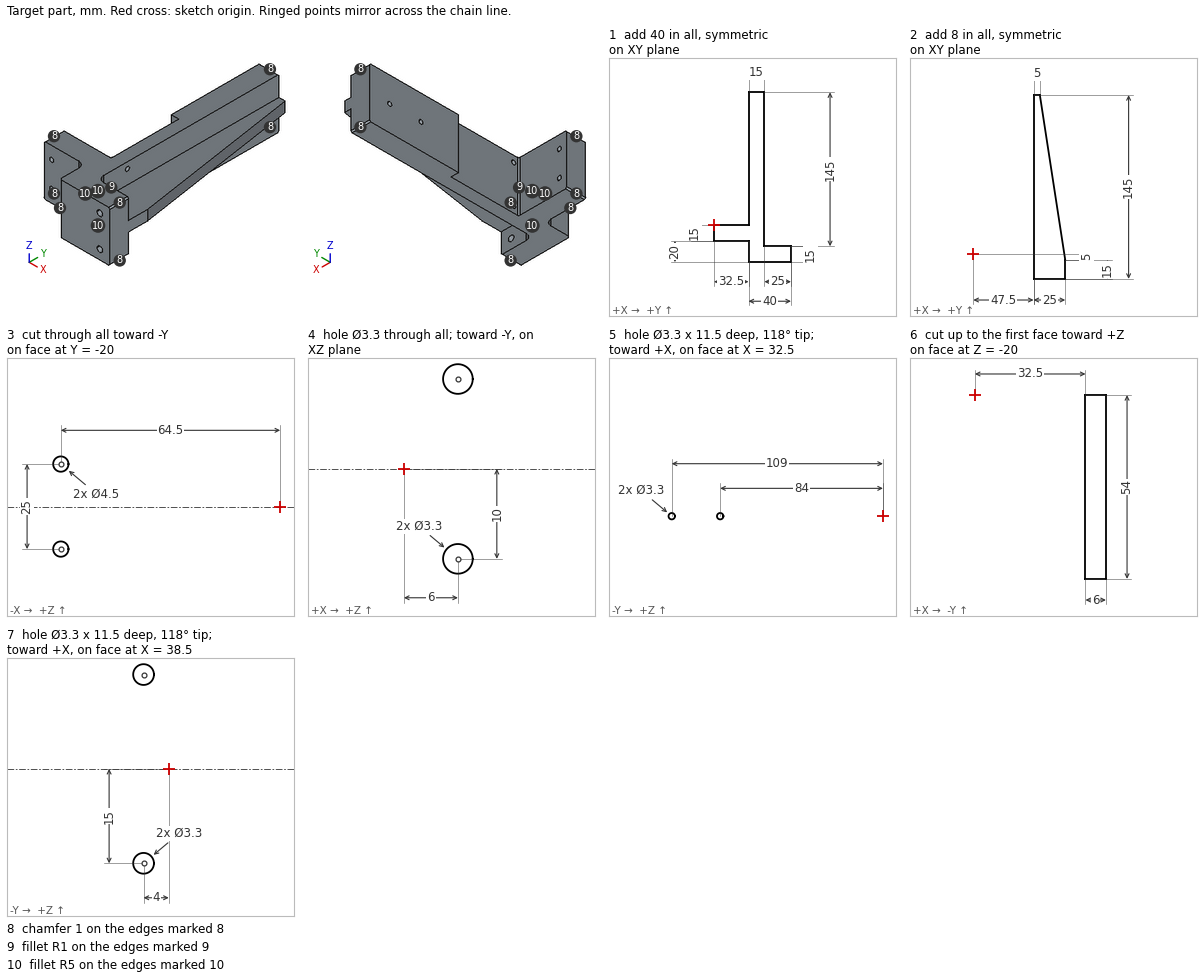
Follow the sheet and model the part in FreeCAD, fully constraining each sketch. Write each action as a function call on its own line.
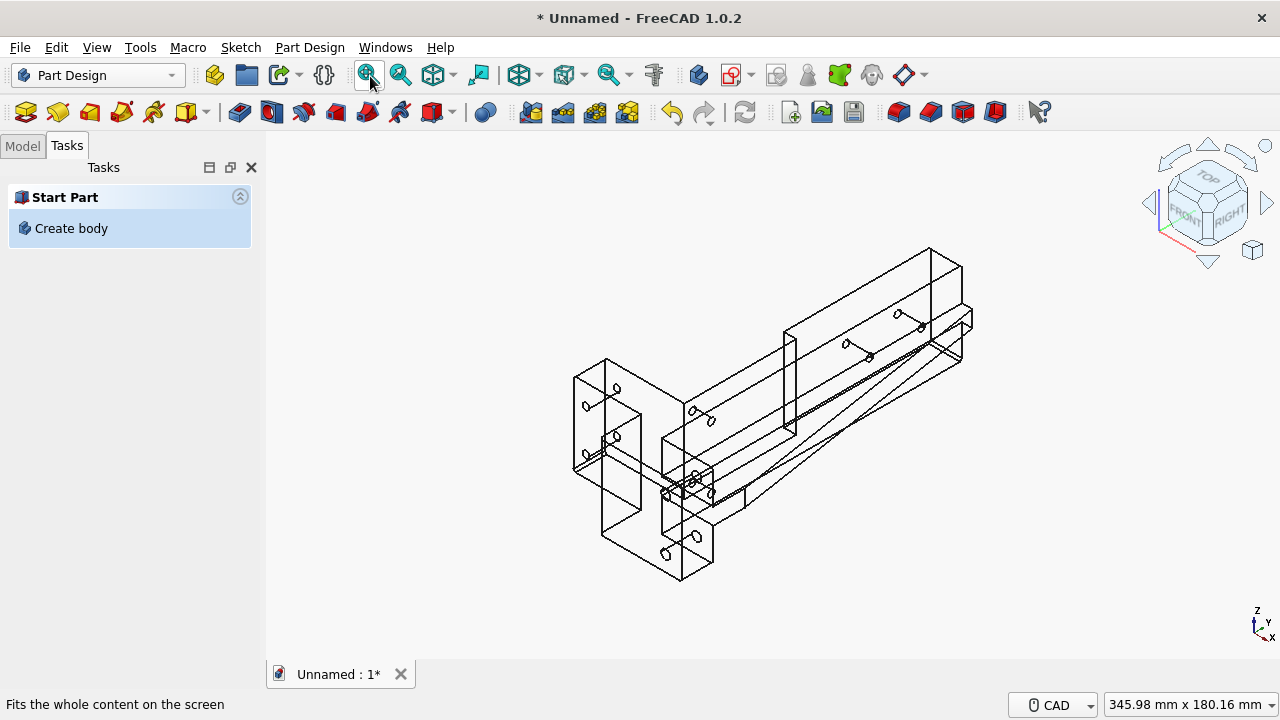
click(684, 441)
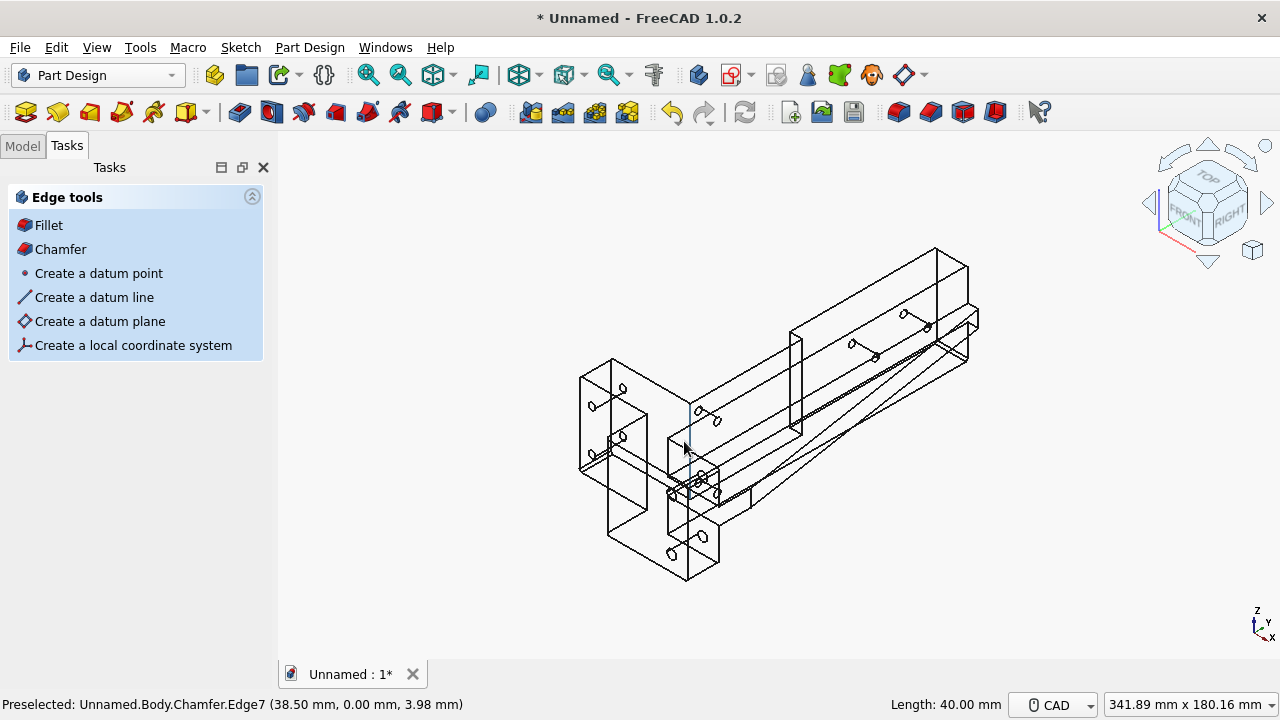
key(v)
key(1)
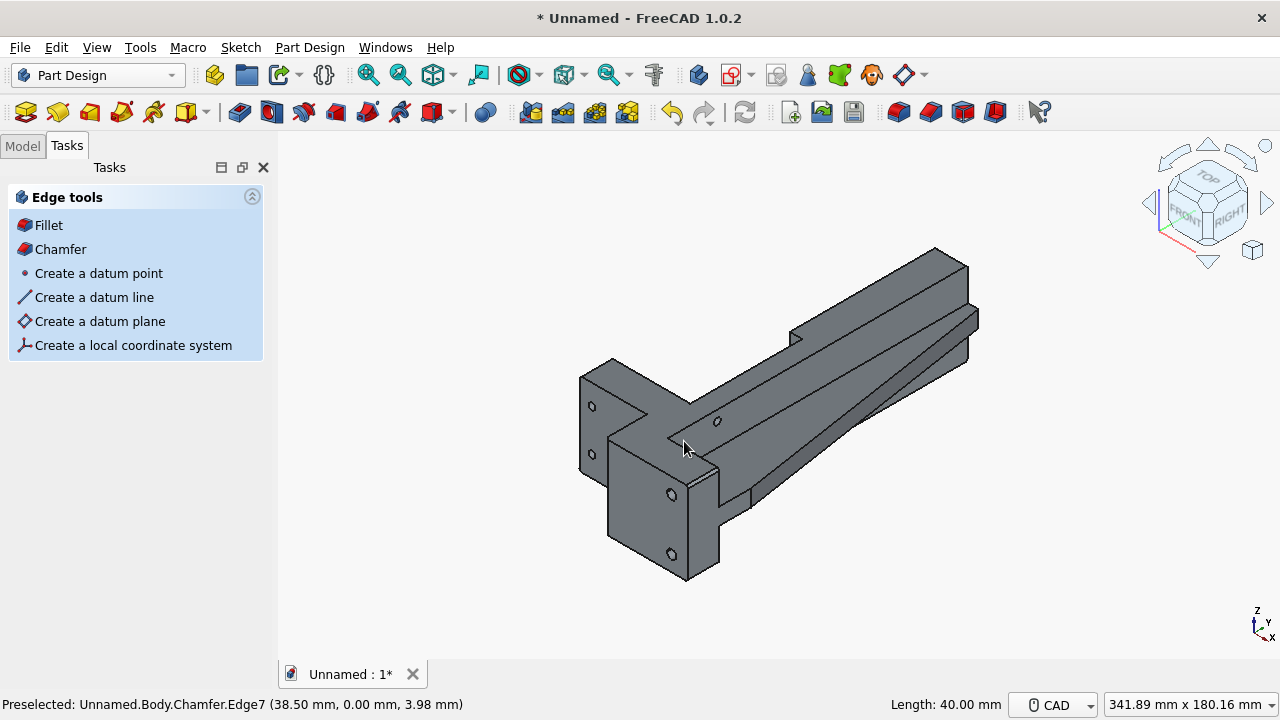
click(900, 112)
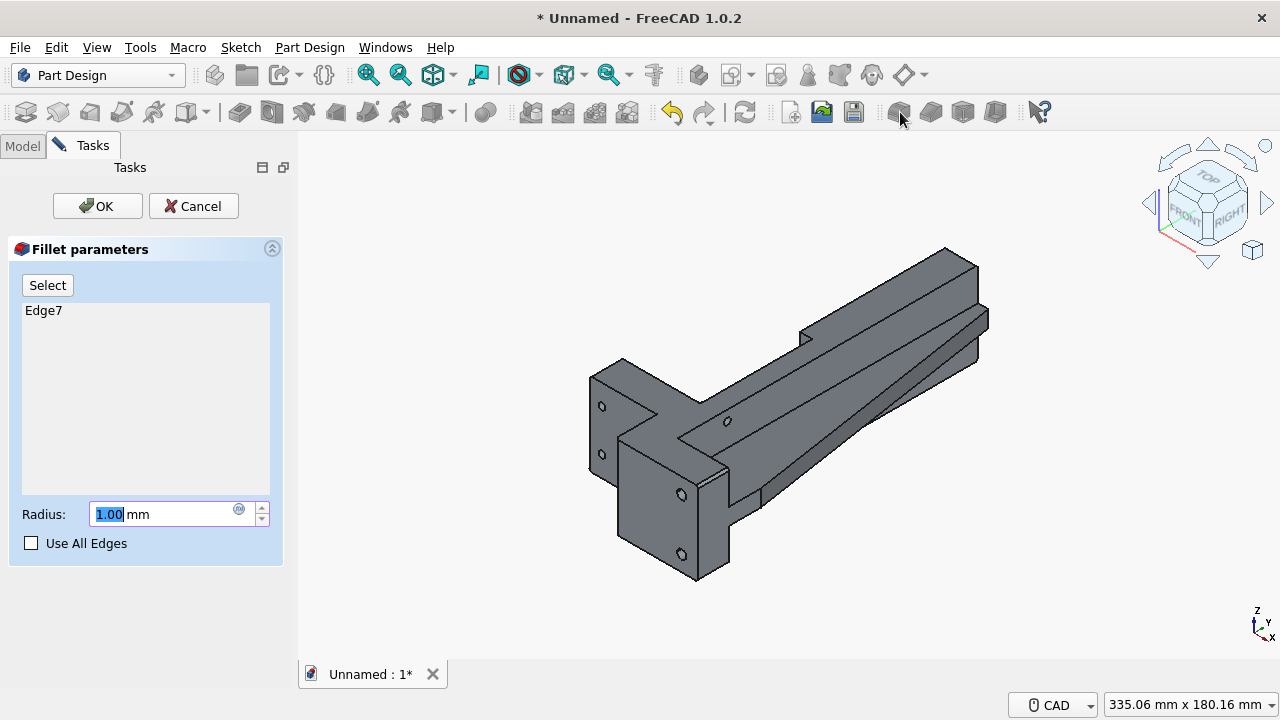
text(1)
key(Tab)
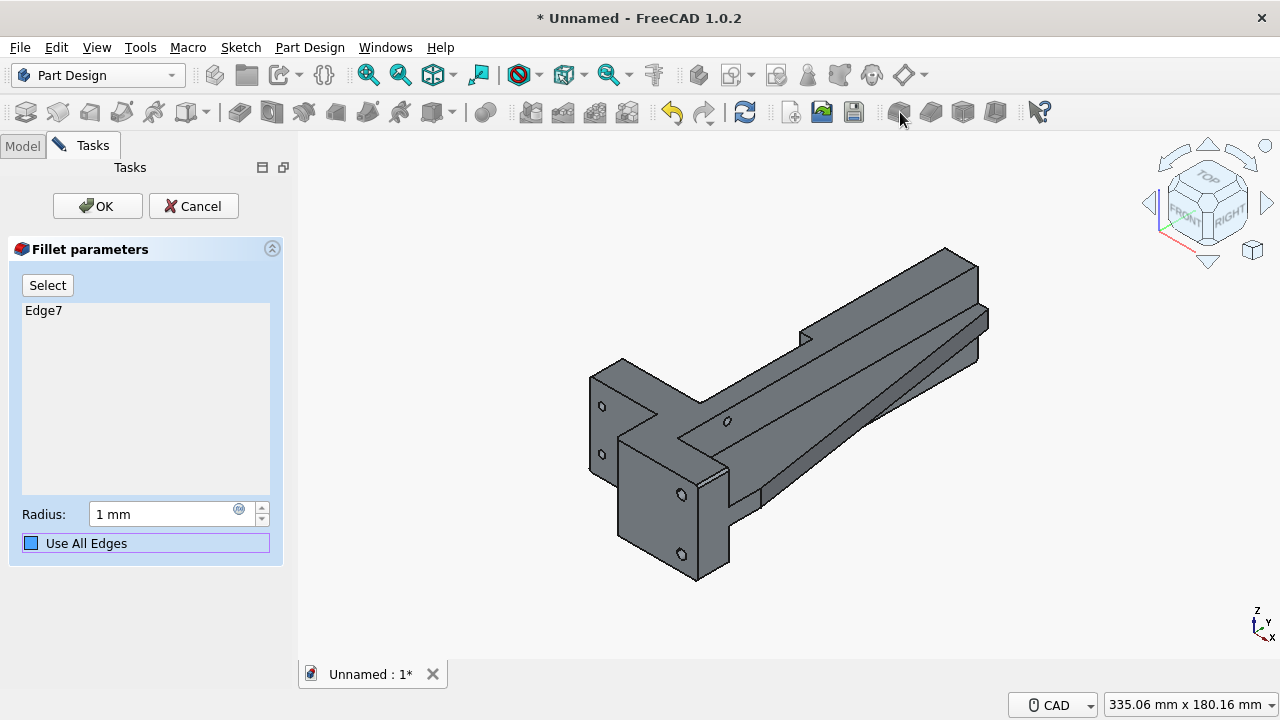
click(98, 206)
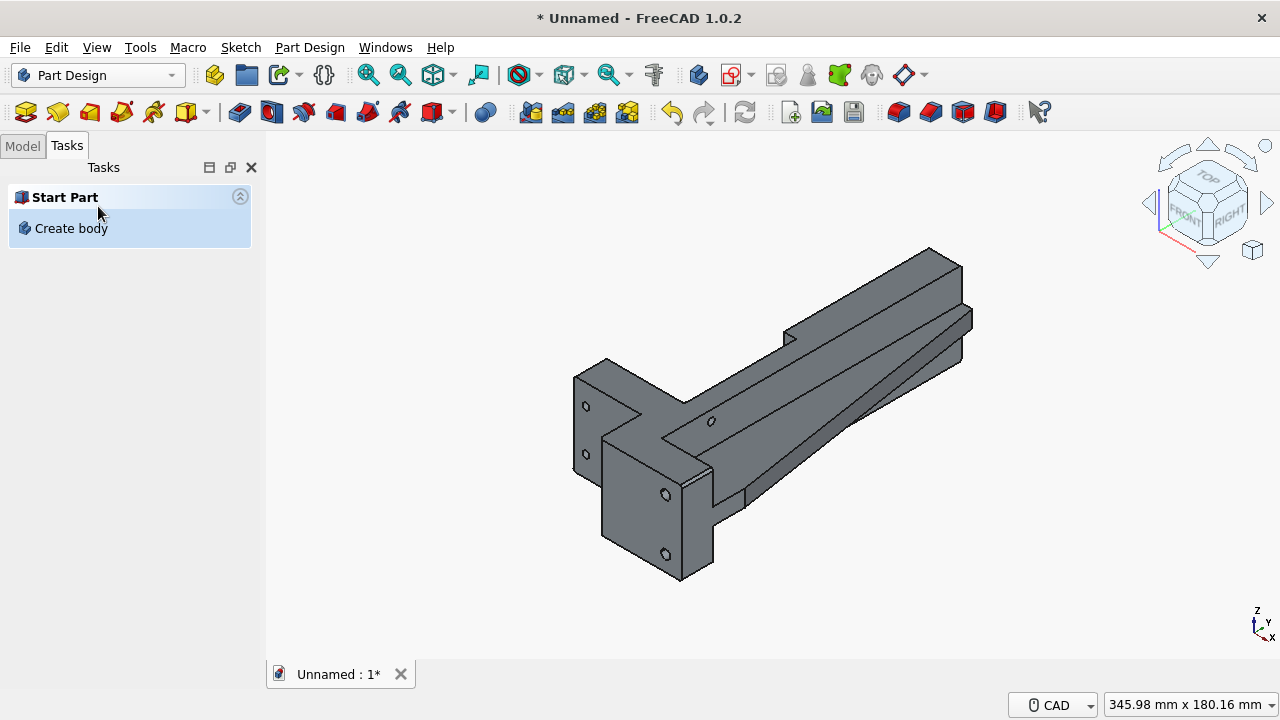
key(2)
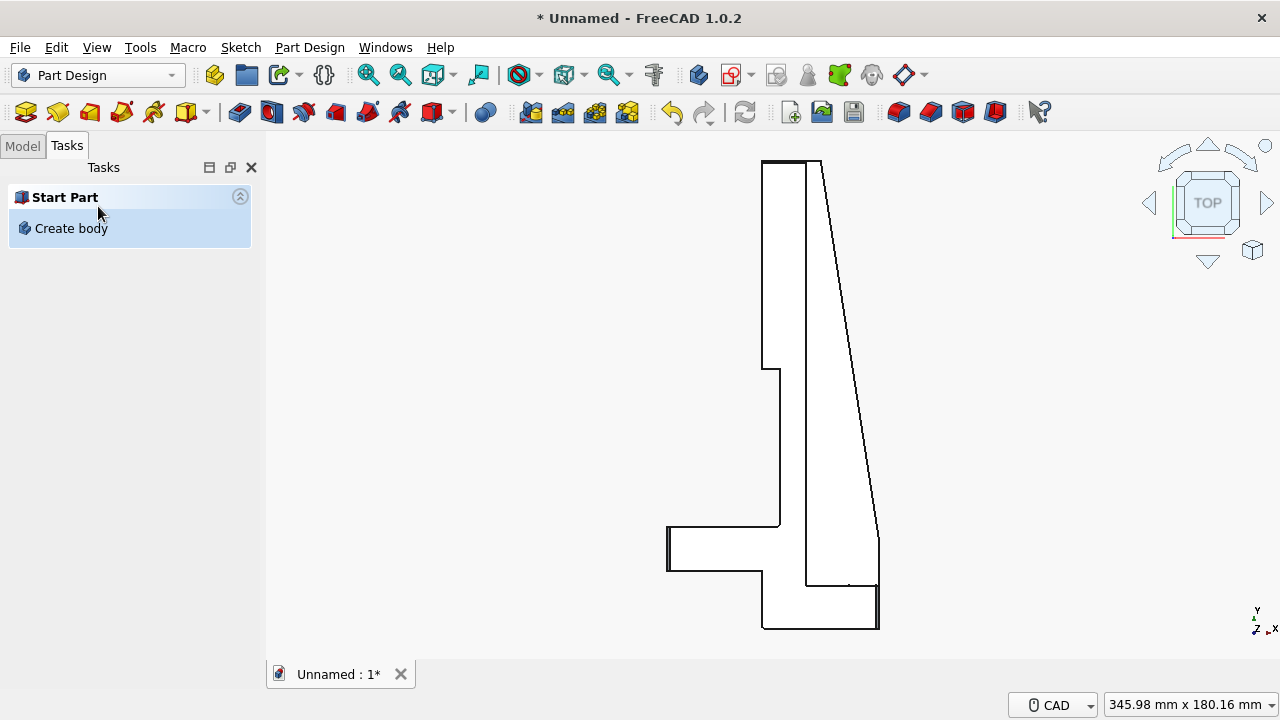
key(0)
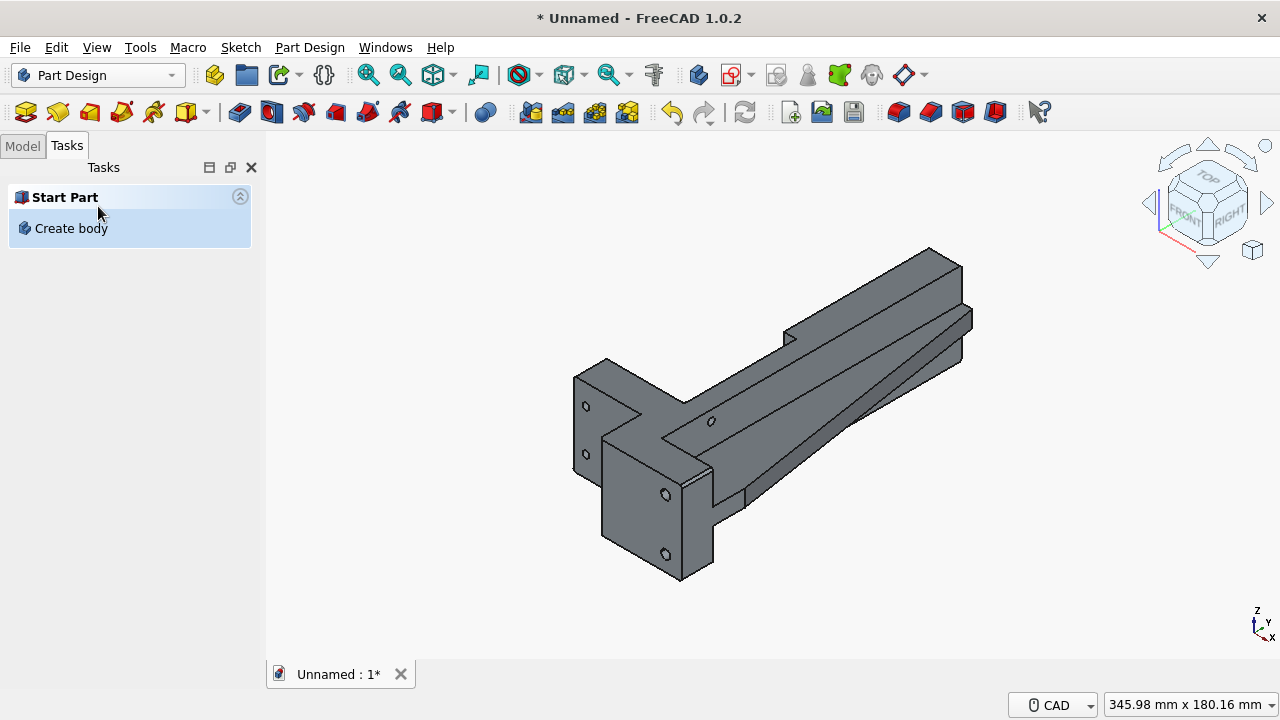
key(1)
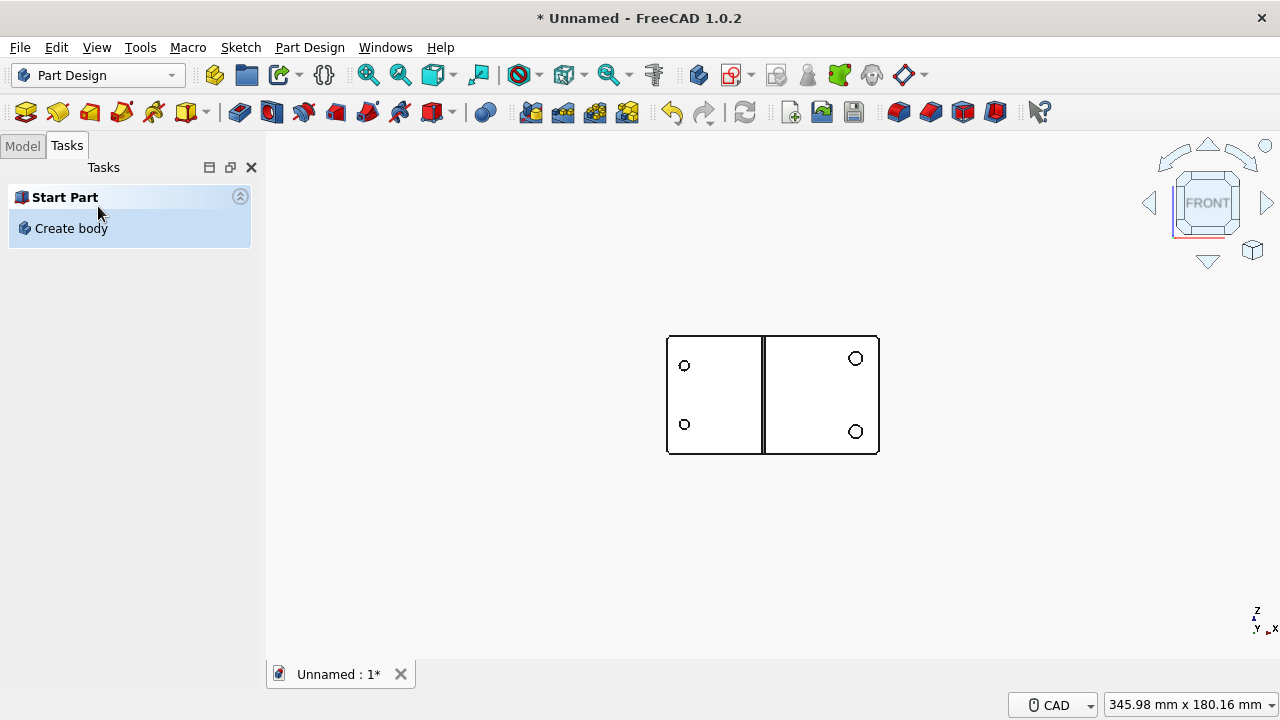
click(370, 76)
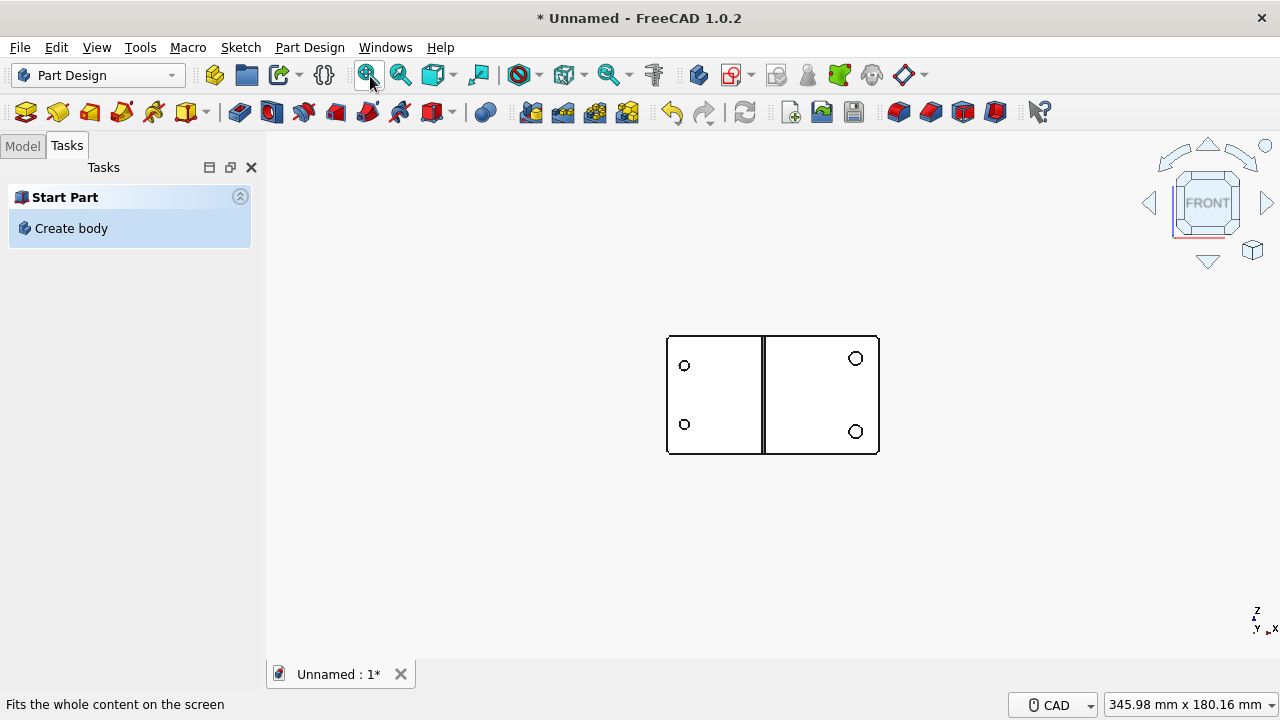
key(3)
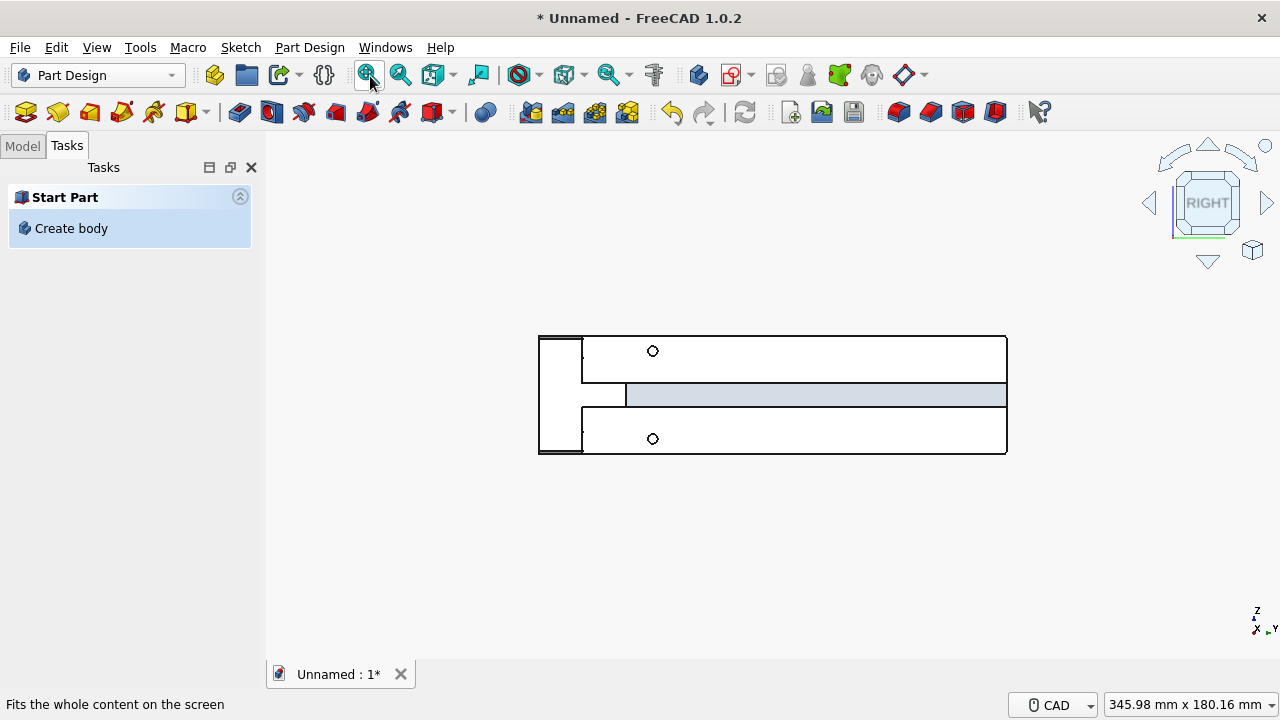
key(5)